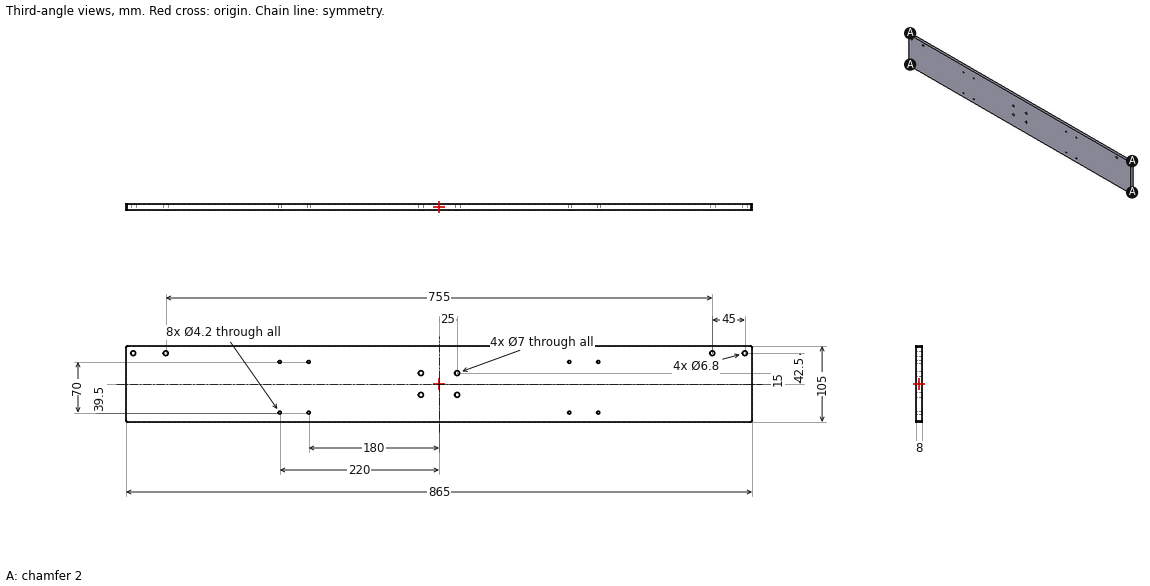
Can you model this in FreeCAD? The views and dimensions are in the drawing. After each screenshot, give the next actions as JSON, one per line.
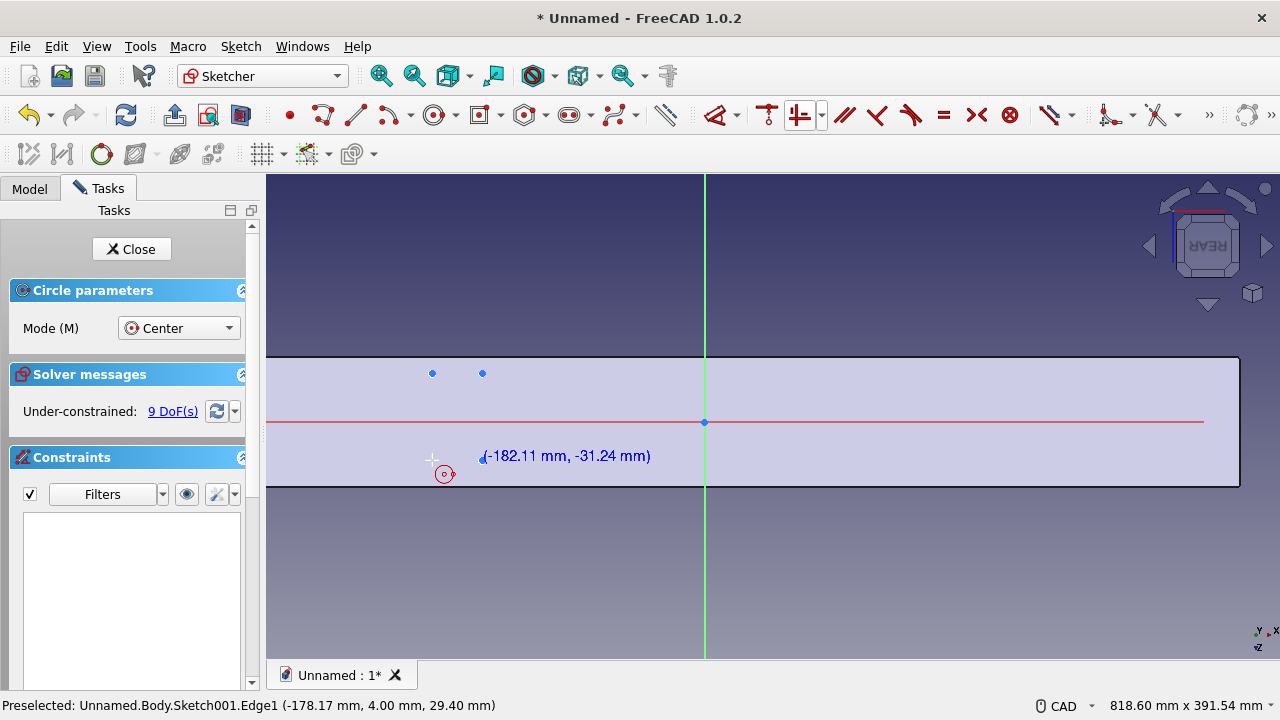
{"action": "left_click", "coordinate": [432, 460]}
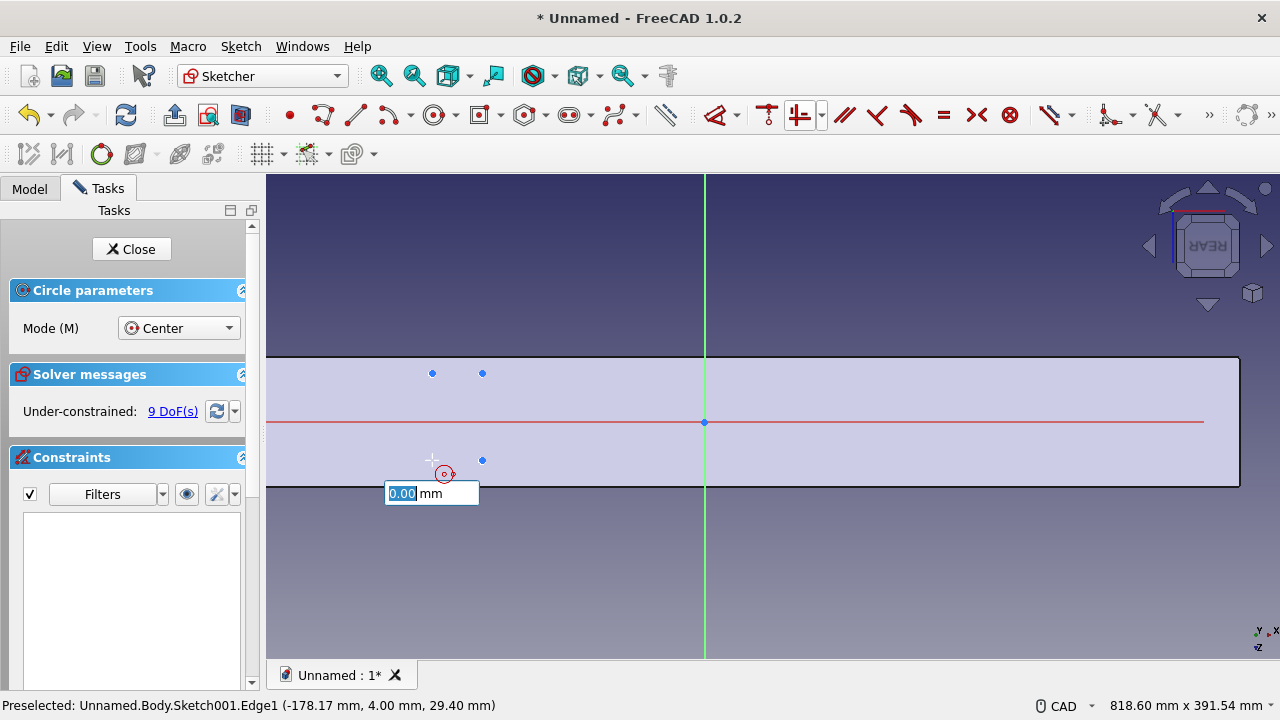
{"action": "scroll", "coordinate": [434, 458], "scroll_direction": "up", "scroll_amount": 10}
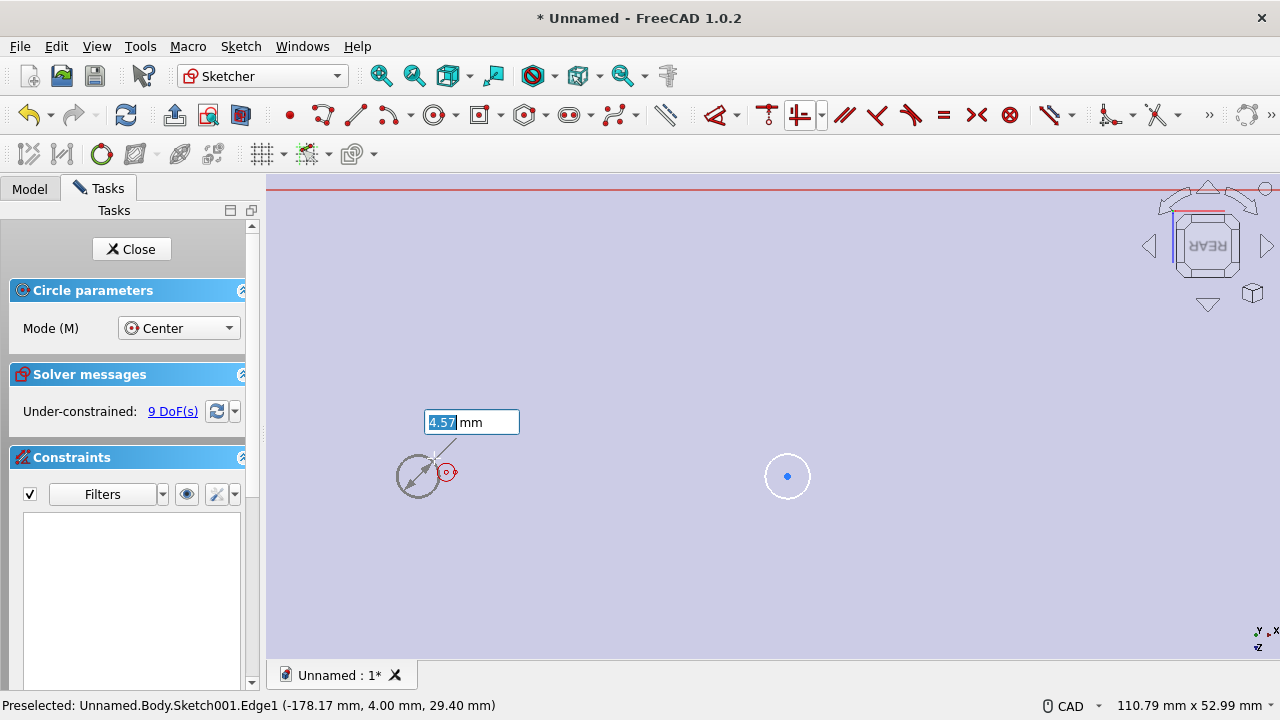
{"action": "left_click", "coordinate": [432, 456]}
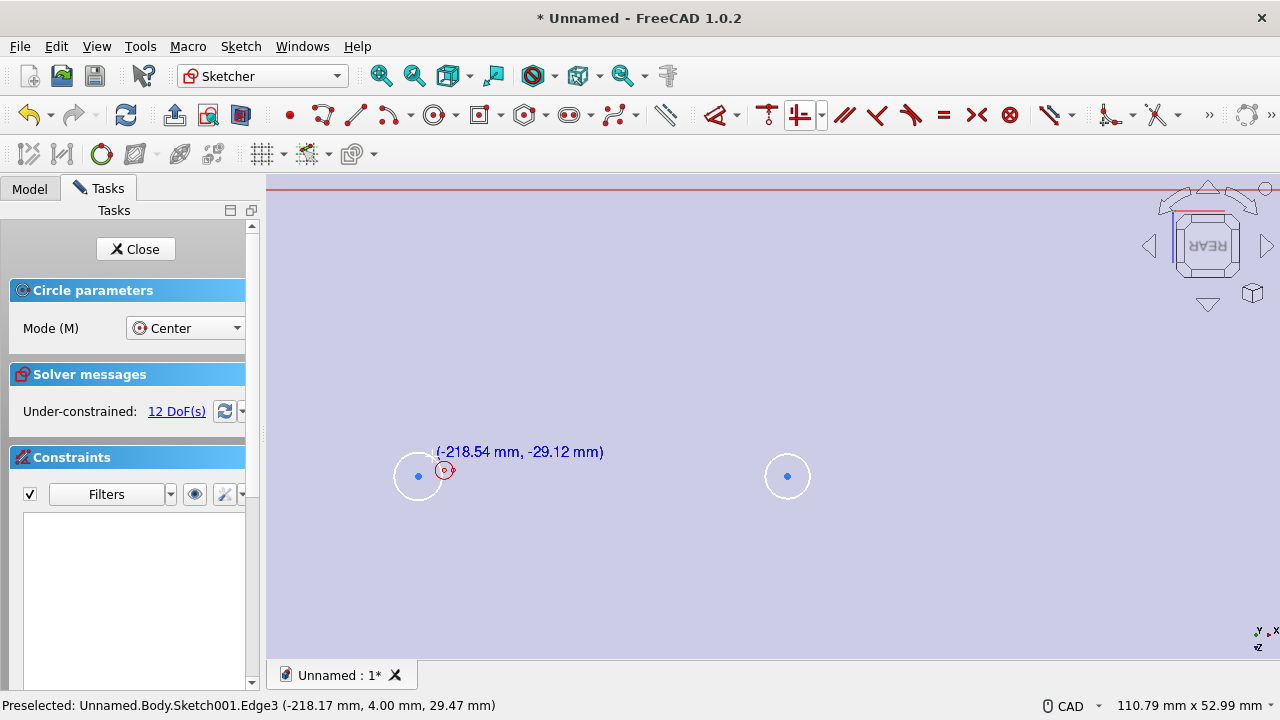
{"action": "scroll", "coordinate": [434, 458], "scroll_direction": "down", "scroll_amount": 10}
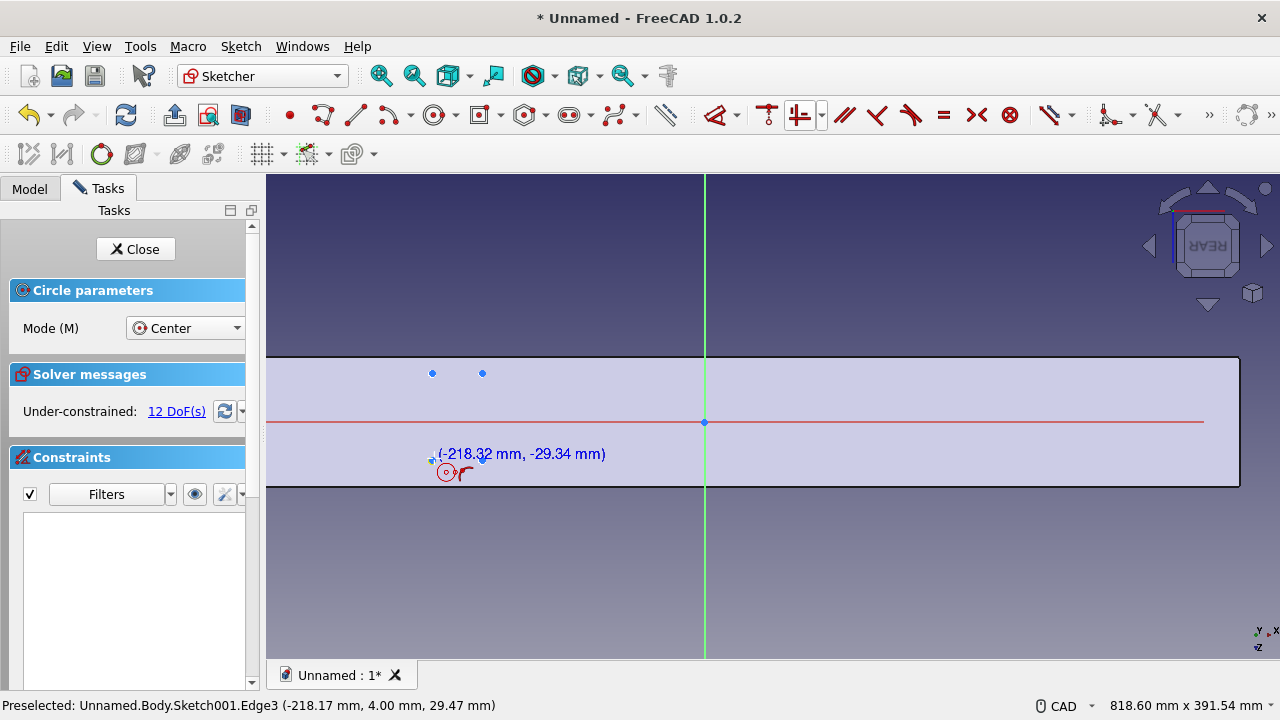
{"action": "scroll", "coordinate": [977, 460], "scroll_direction": "up", "scroll_amount": 11}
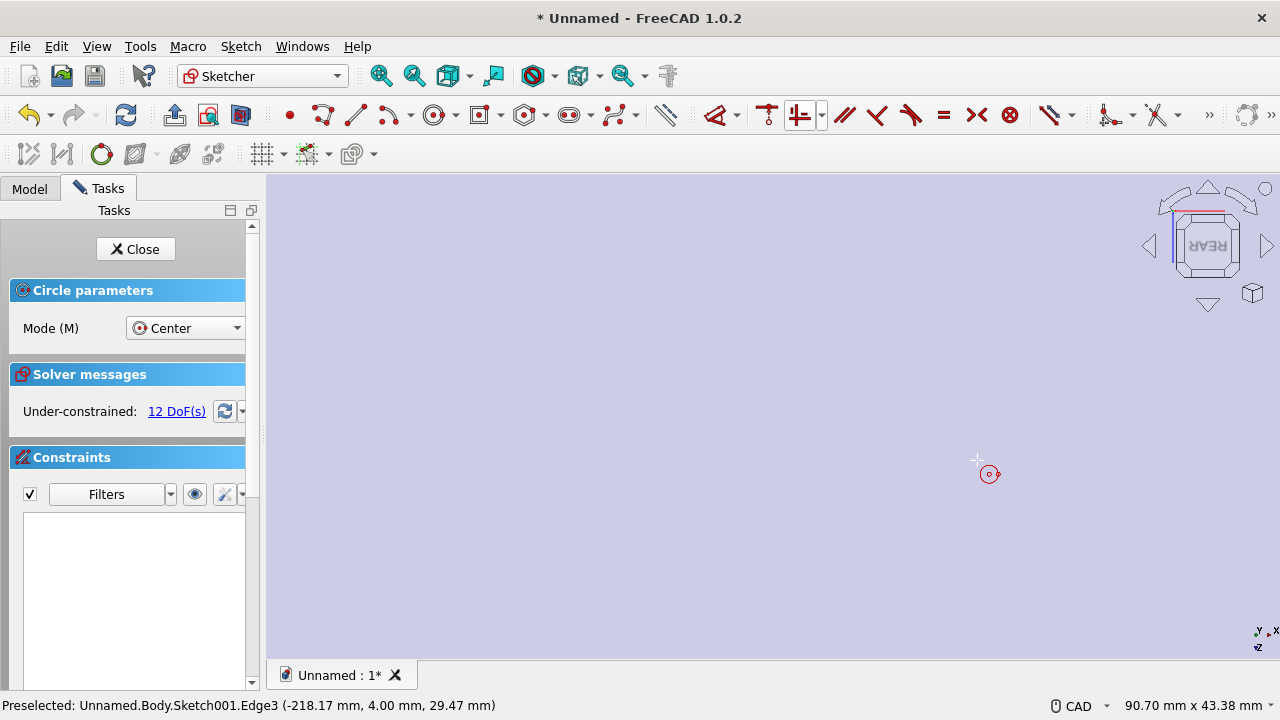
{"action": "scroll", "coordinate": [978, 460], "scroll_direction": "down", "scroll_amount": 11}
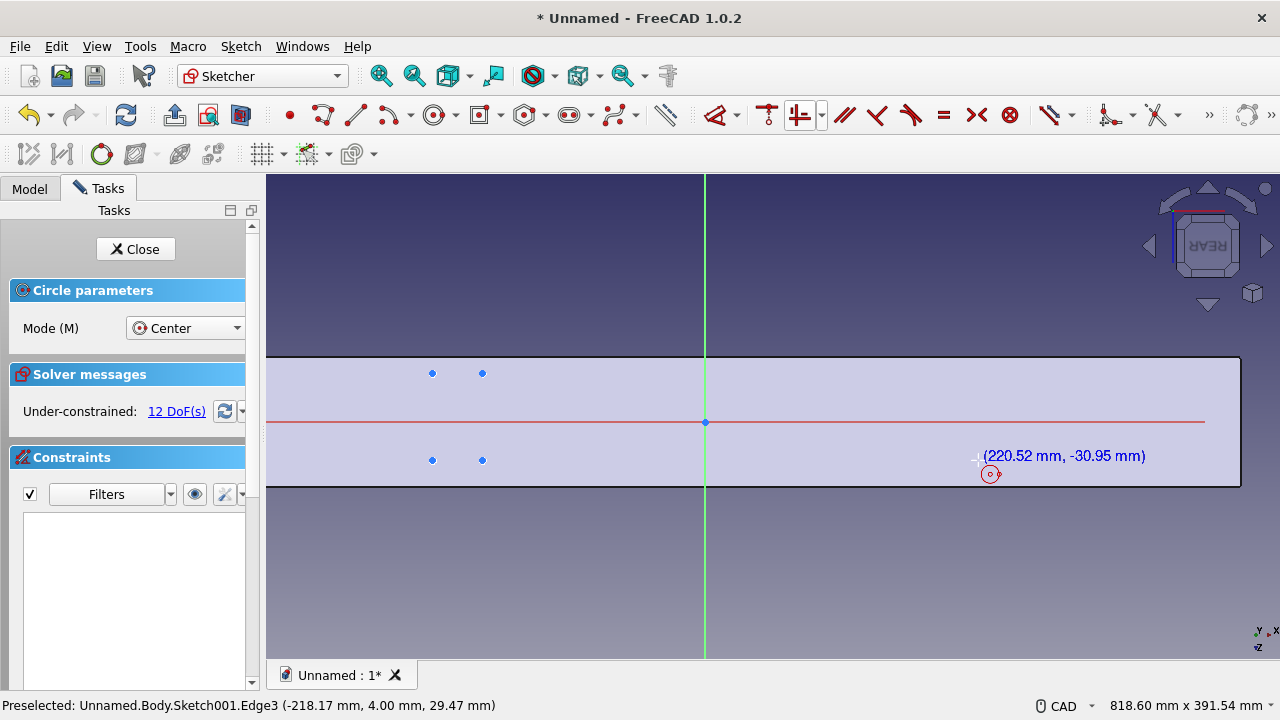
{"action": "left_click", "coordinate": [978, 460]}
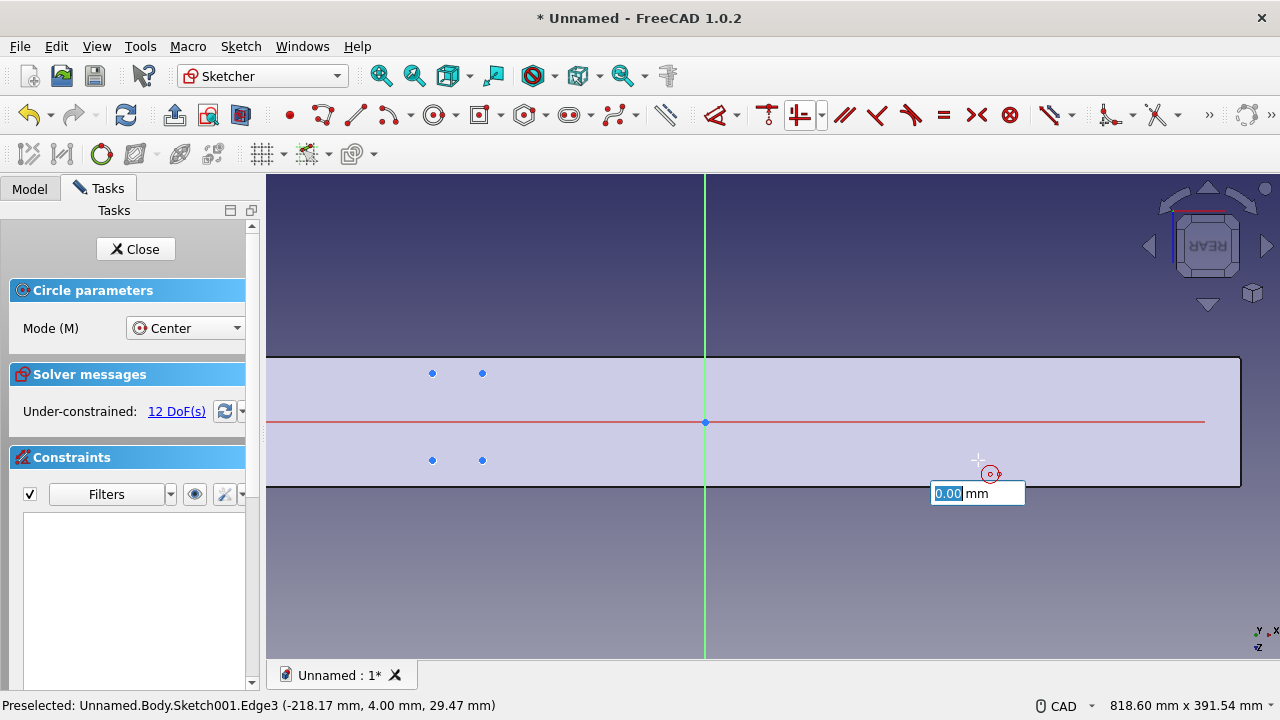
{"action": "scroll", "coordinate": [980, 458], "scroll_direction": "up", "scroll_amount": 10}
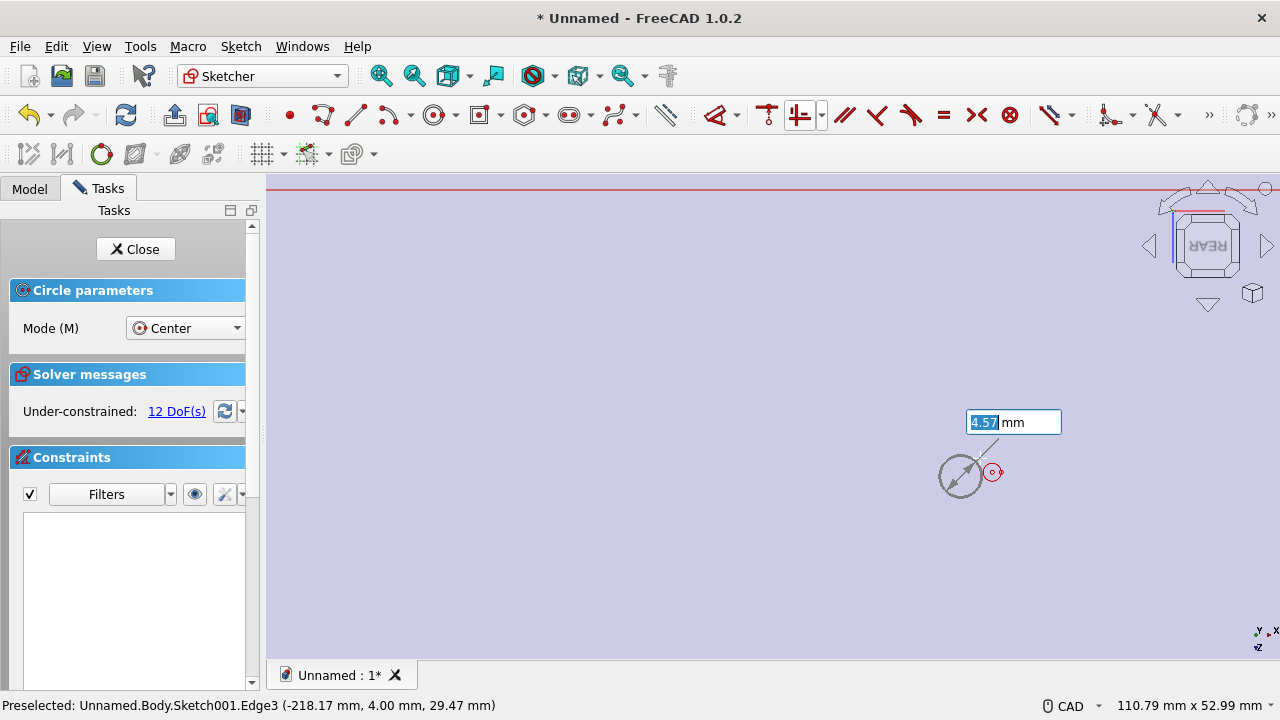
{"action": "left_click", "coordinate": [974, 456]}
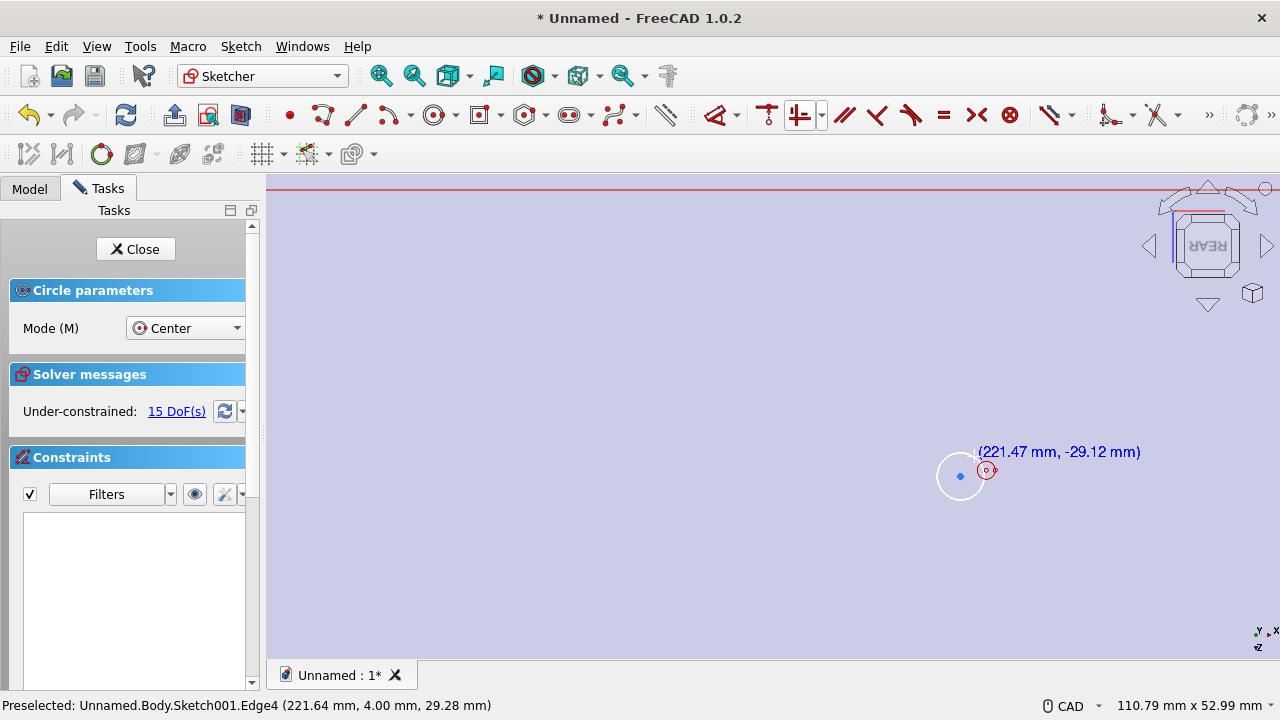
{"action": "scroll", "coordinate": [980, 458], "scroll_direction": "down", "scroll_amount": 10}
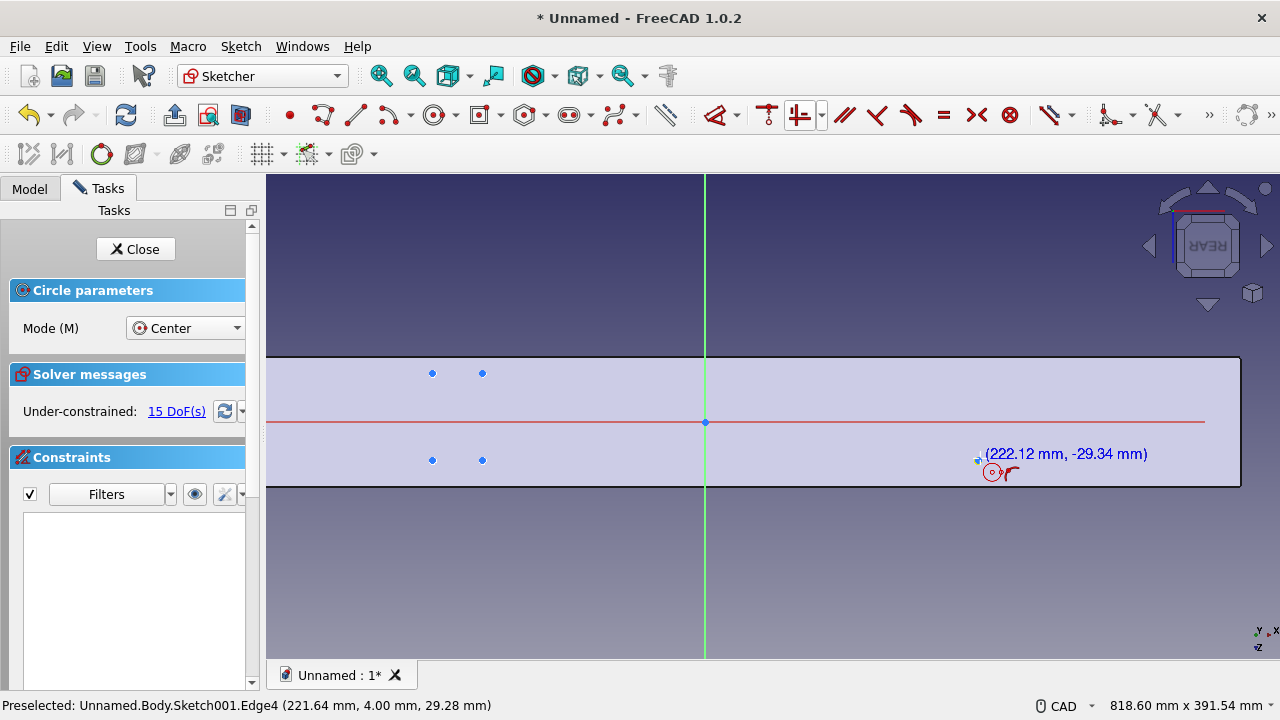
{"action": "left_click", "coordinate": [928, 460]}